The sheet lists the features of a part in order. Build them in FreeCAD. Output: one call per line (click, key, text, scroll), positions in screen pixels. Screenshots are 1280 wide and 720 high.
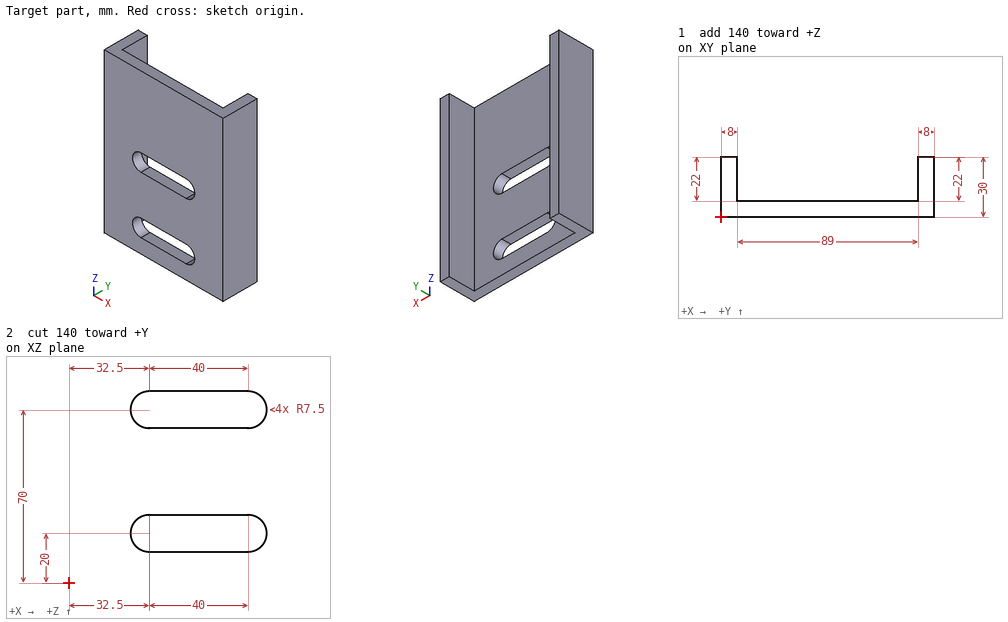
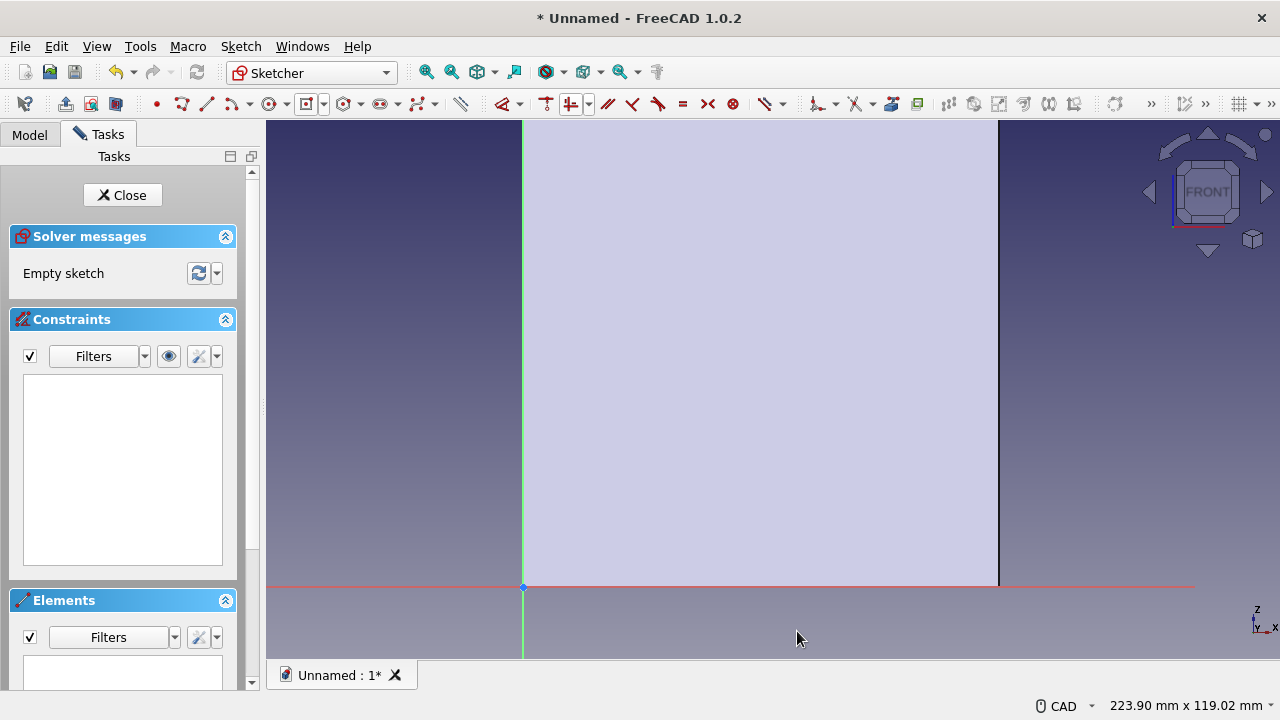
click(380, 104)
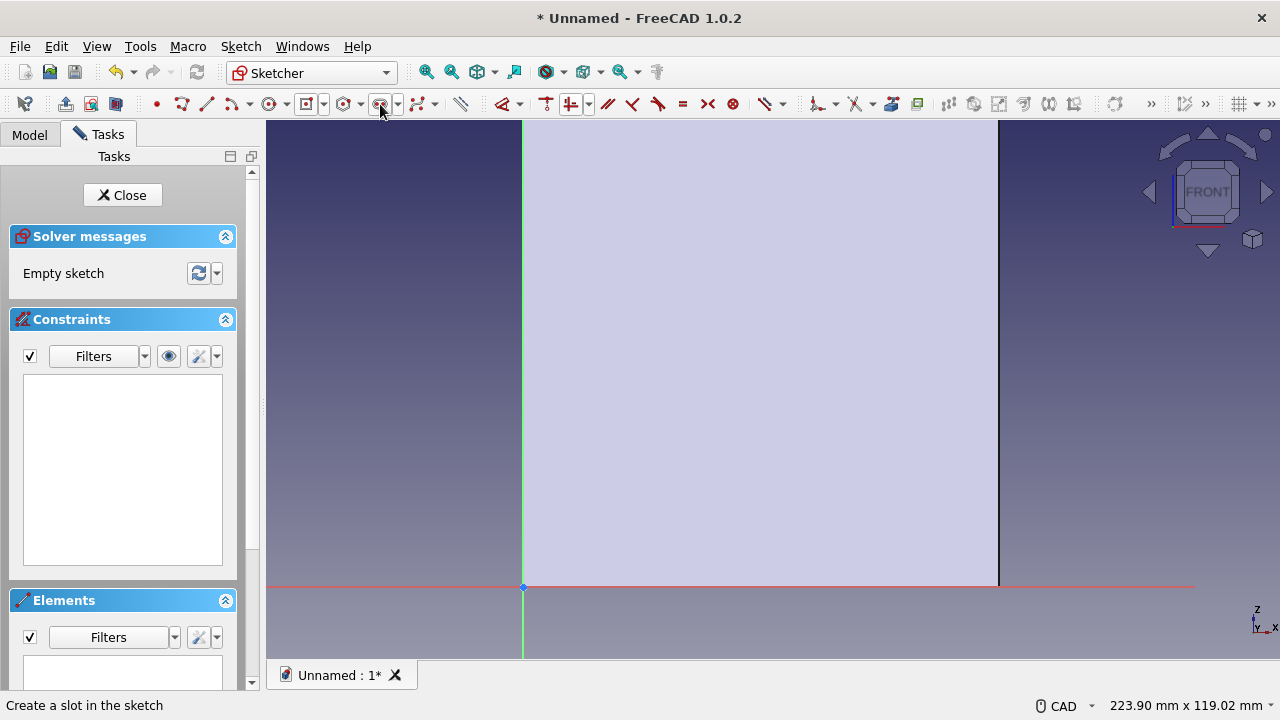
click(670, 270)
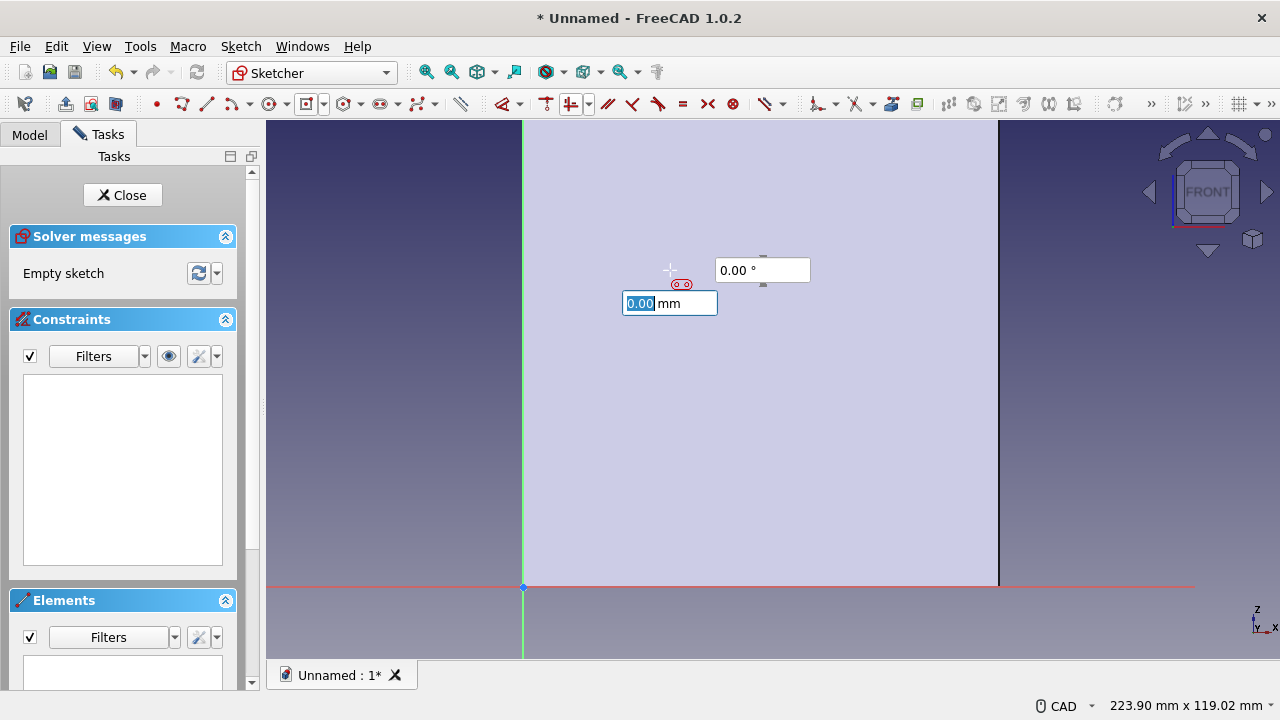
click(852, 270)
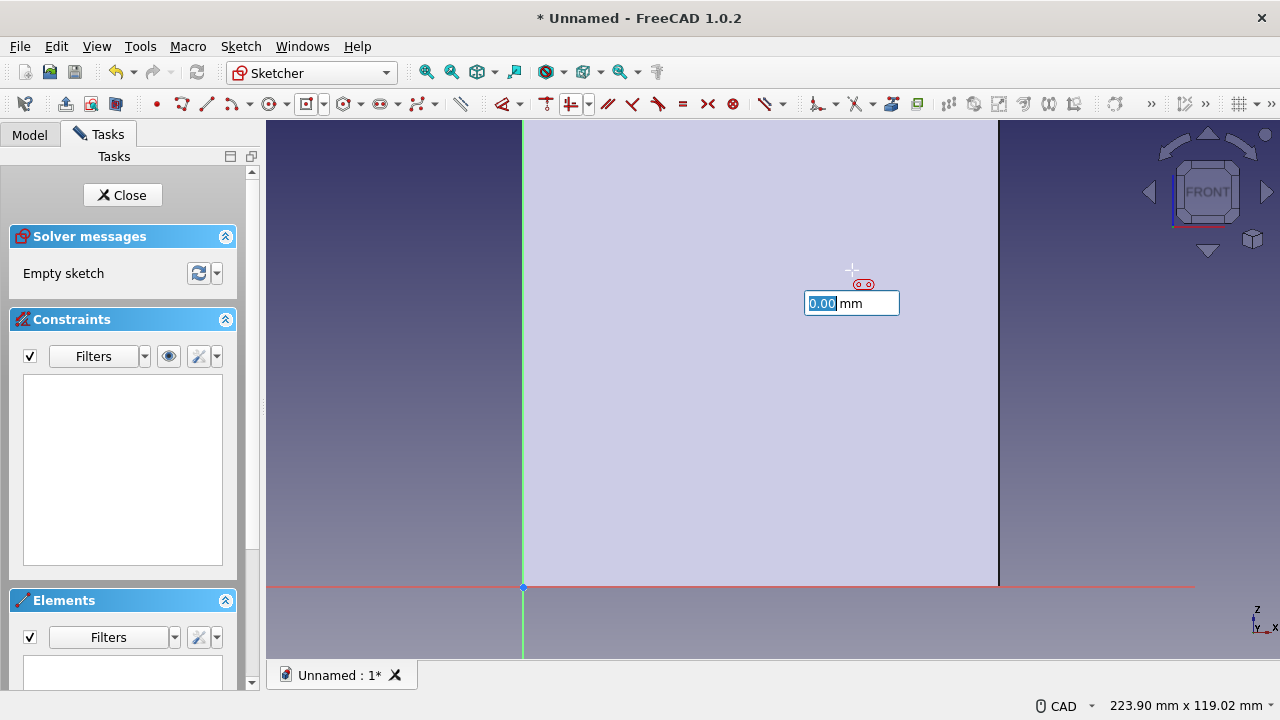
click(761, 236)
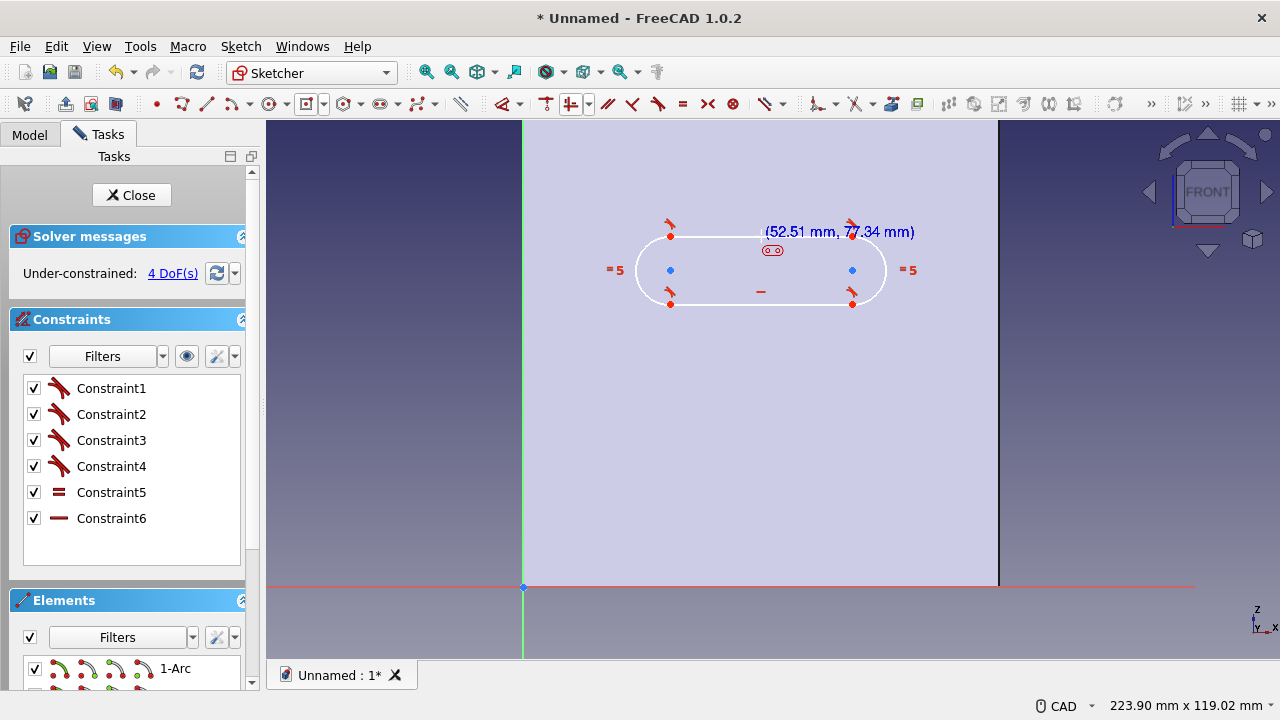
click(670, 497)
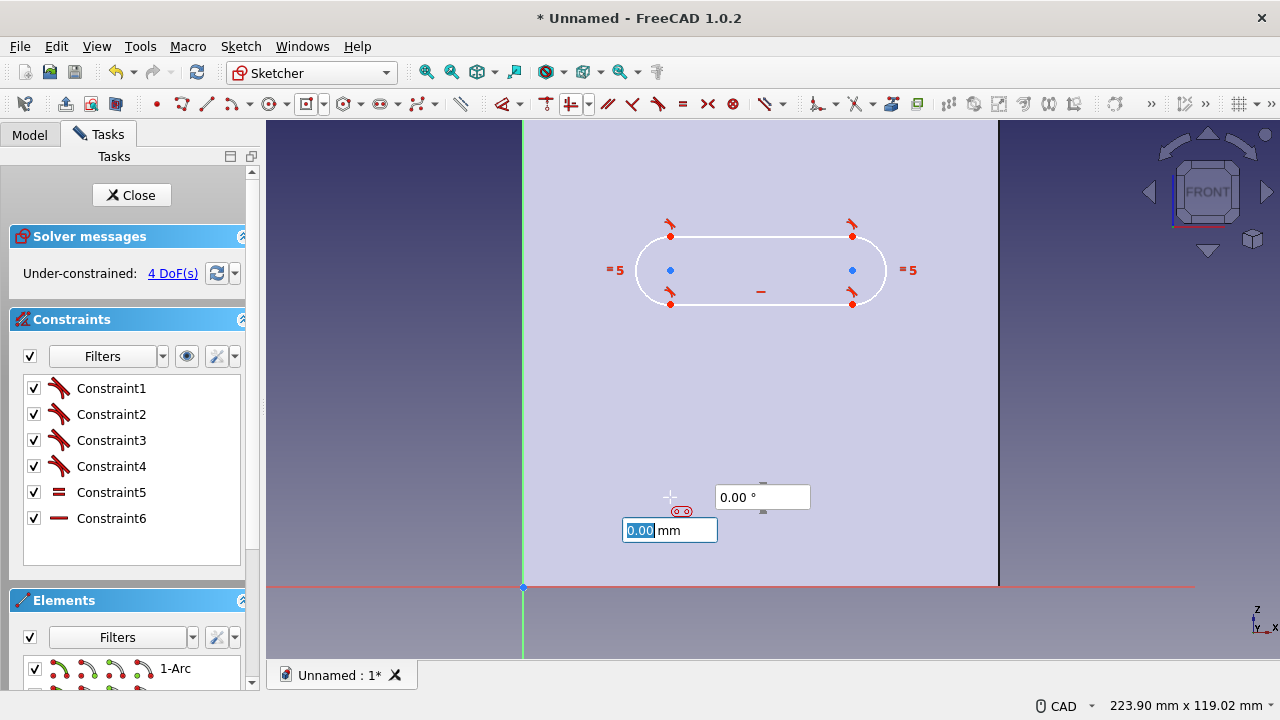
click(852, 497)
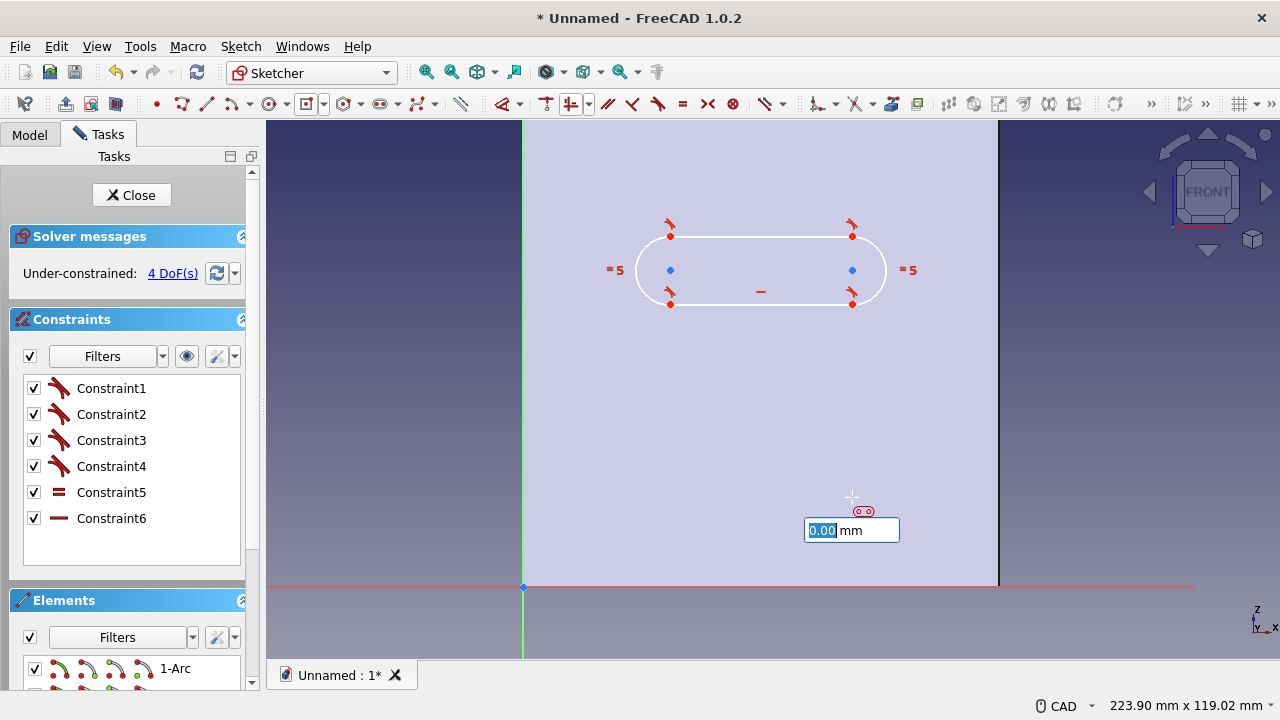
click(761, 531)
key(Escape)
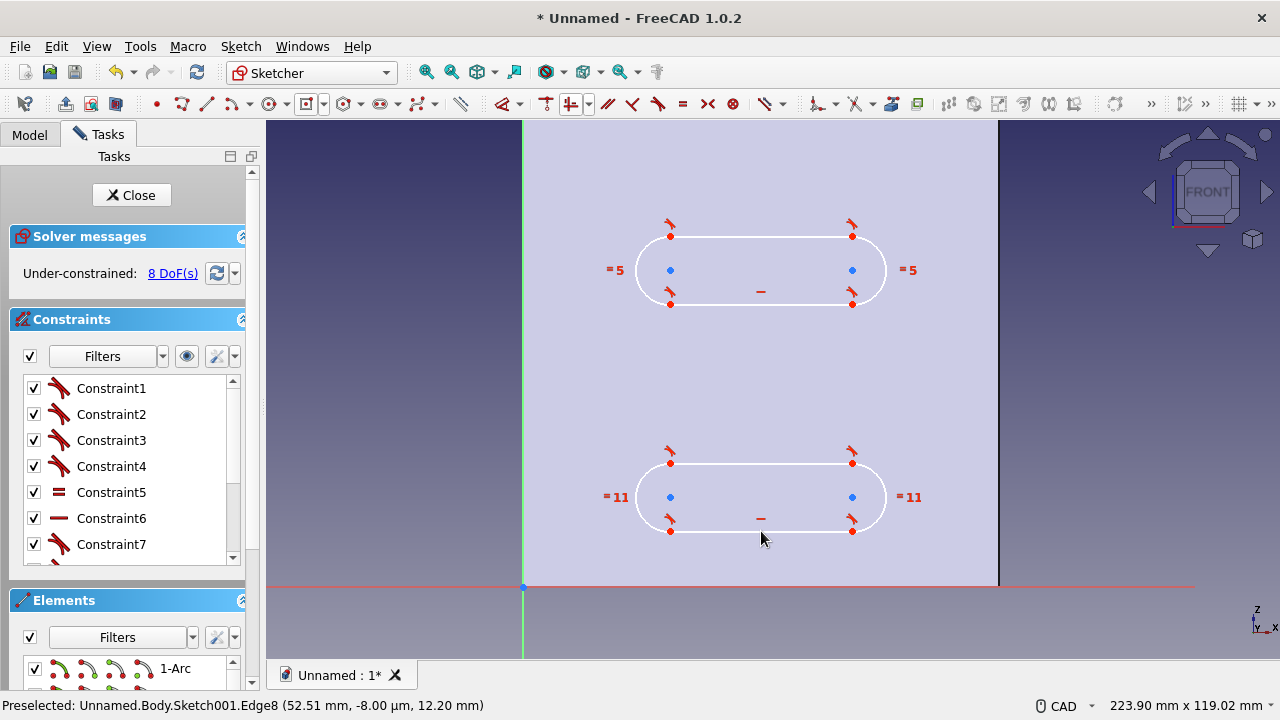
click(642, 251)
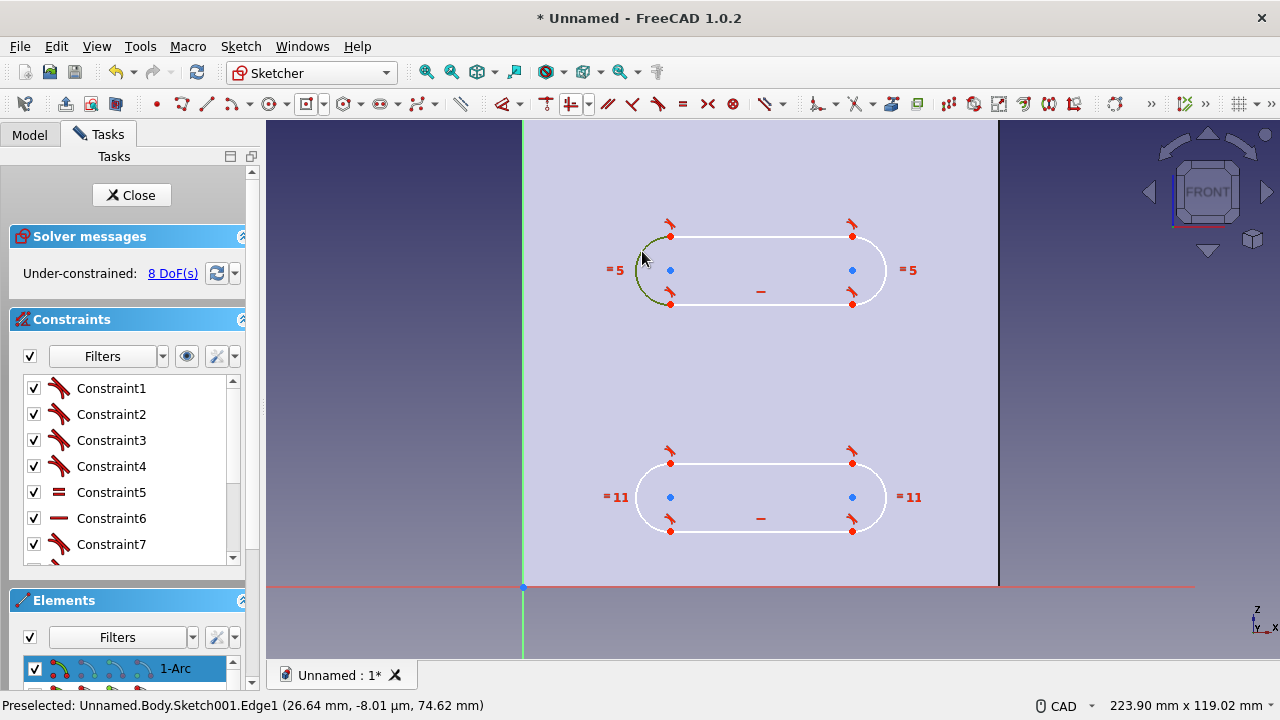
click(642, 478)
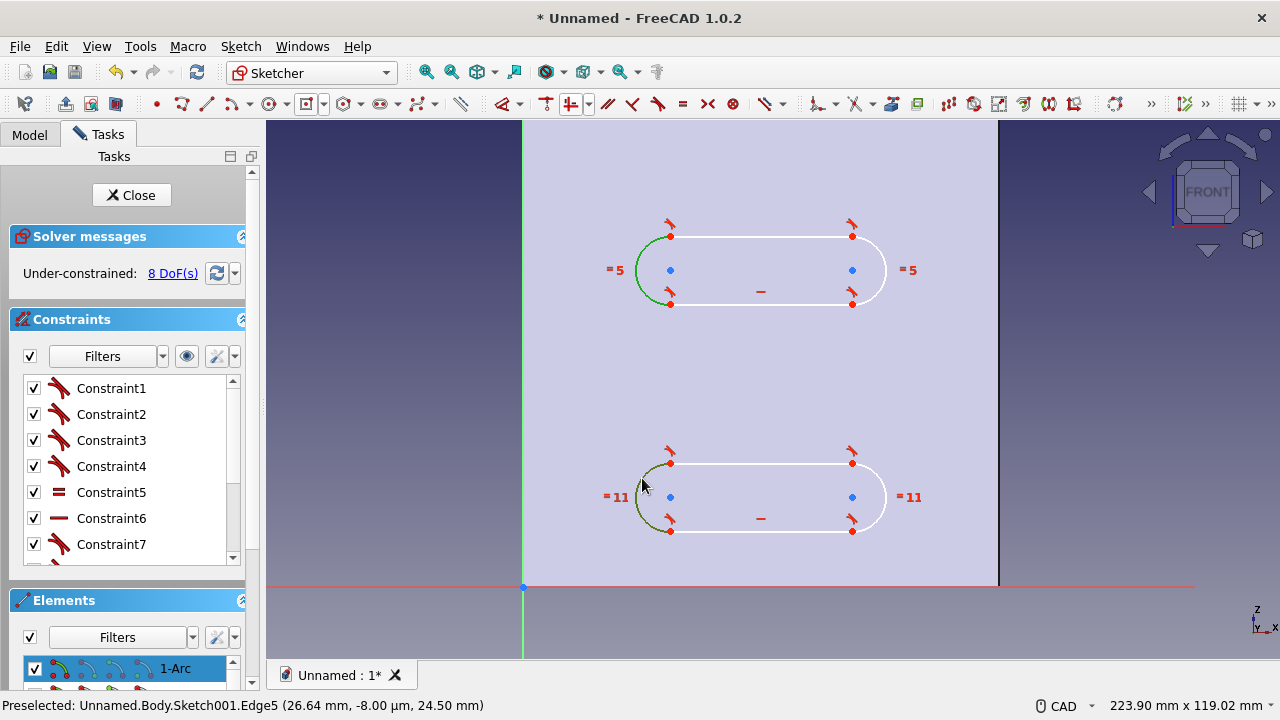
click(683, 104)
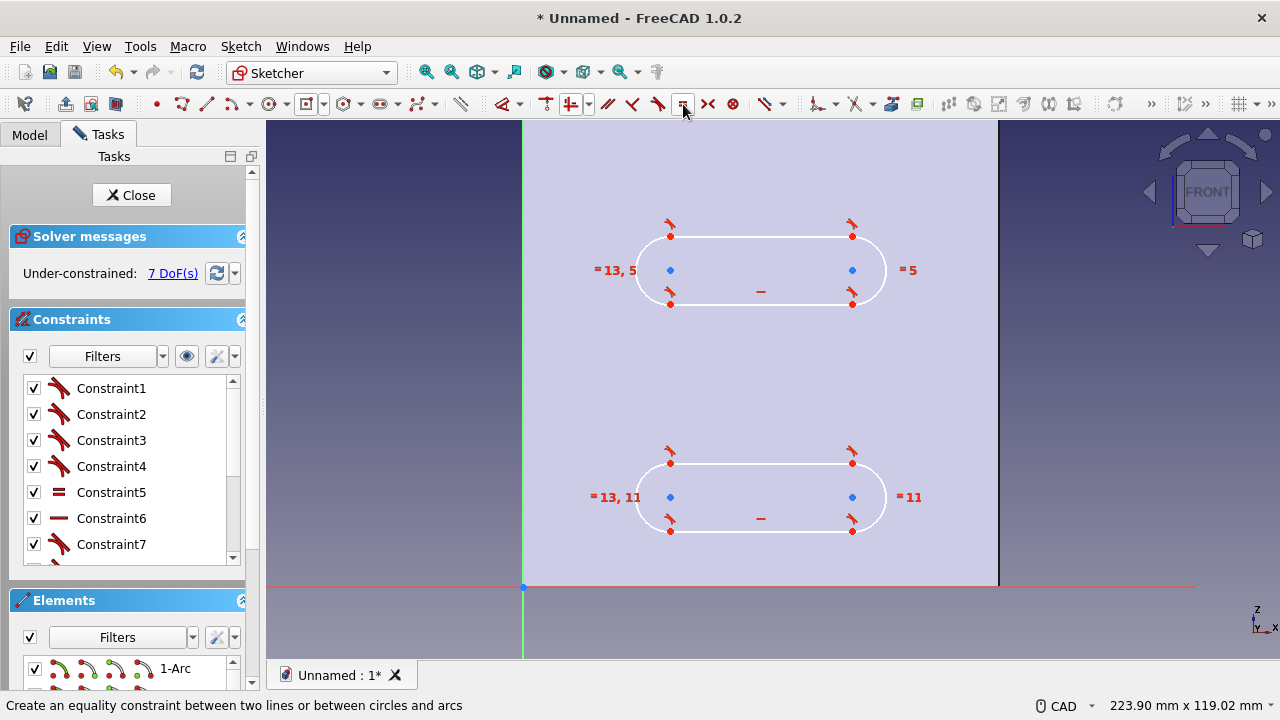
click(502, 104)